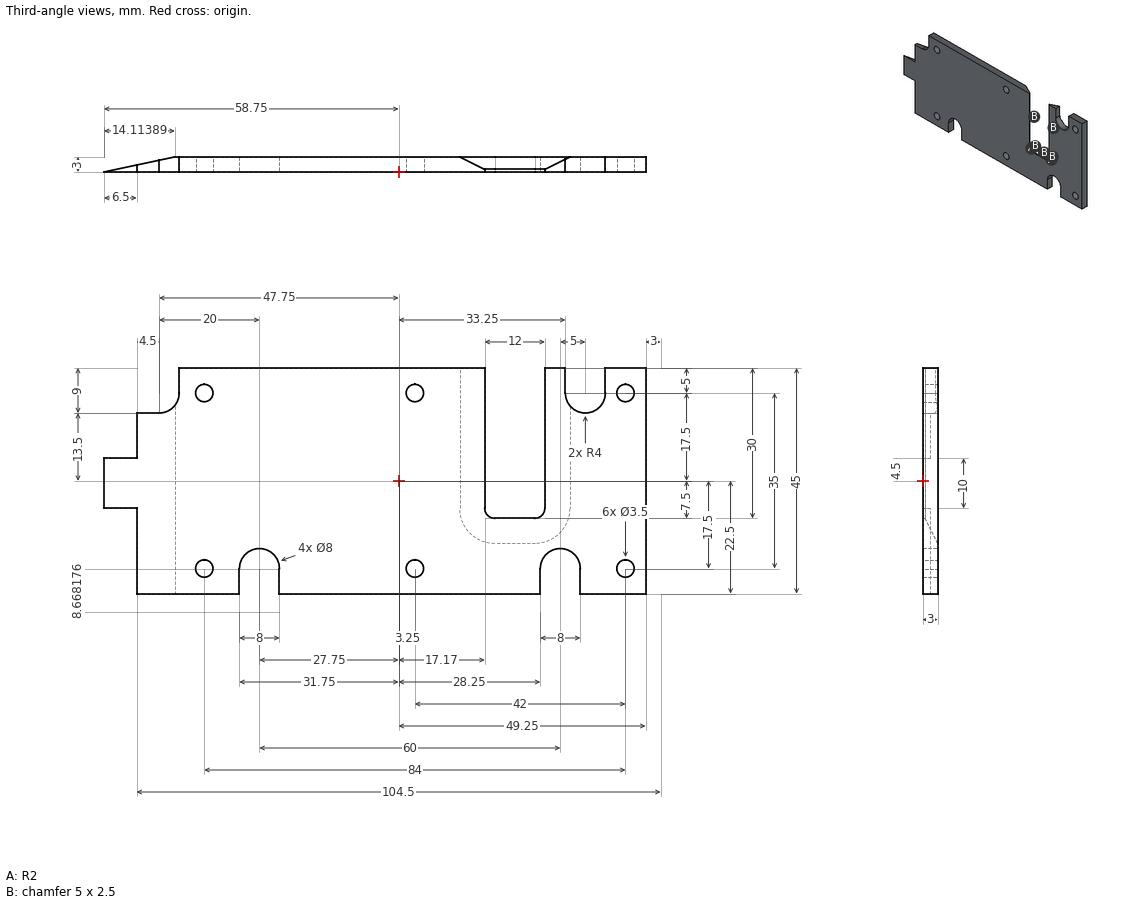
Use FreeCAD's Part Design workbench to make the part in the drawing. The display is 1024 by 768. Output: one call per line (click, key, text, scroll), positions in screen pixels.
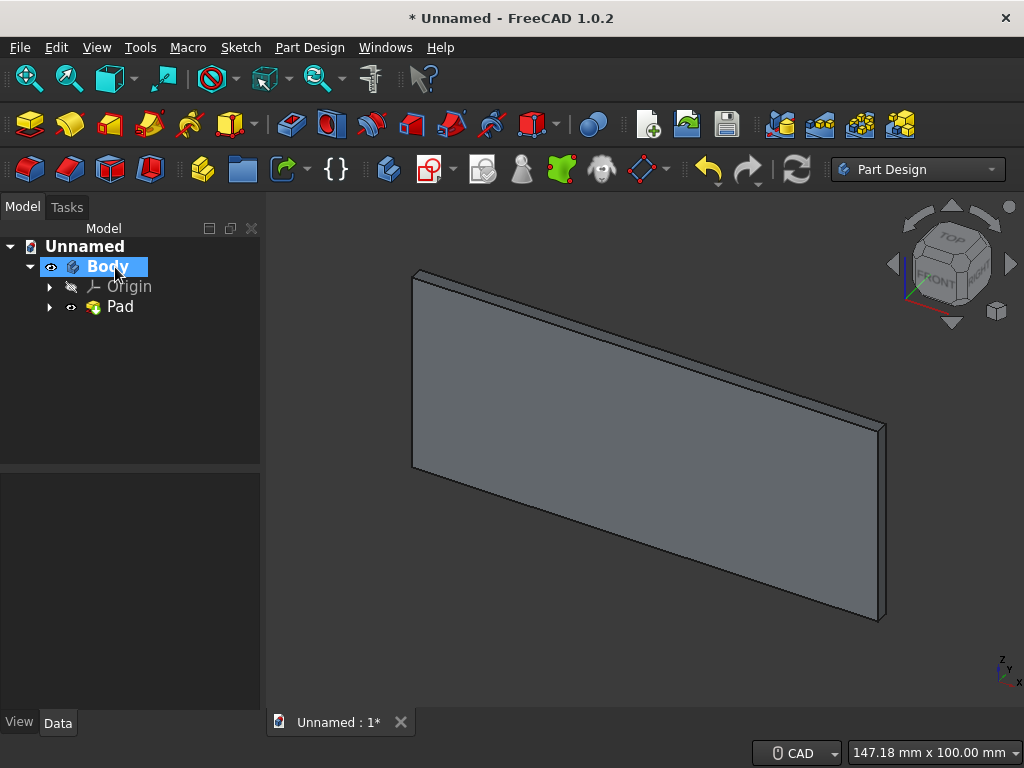
key(4)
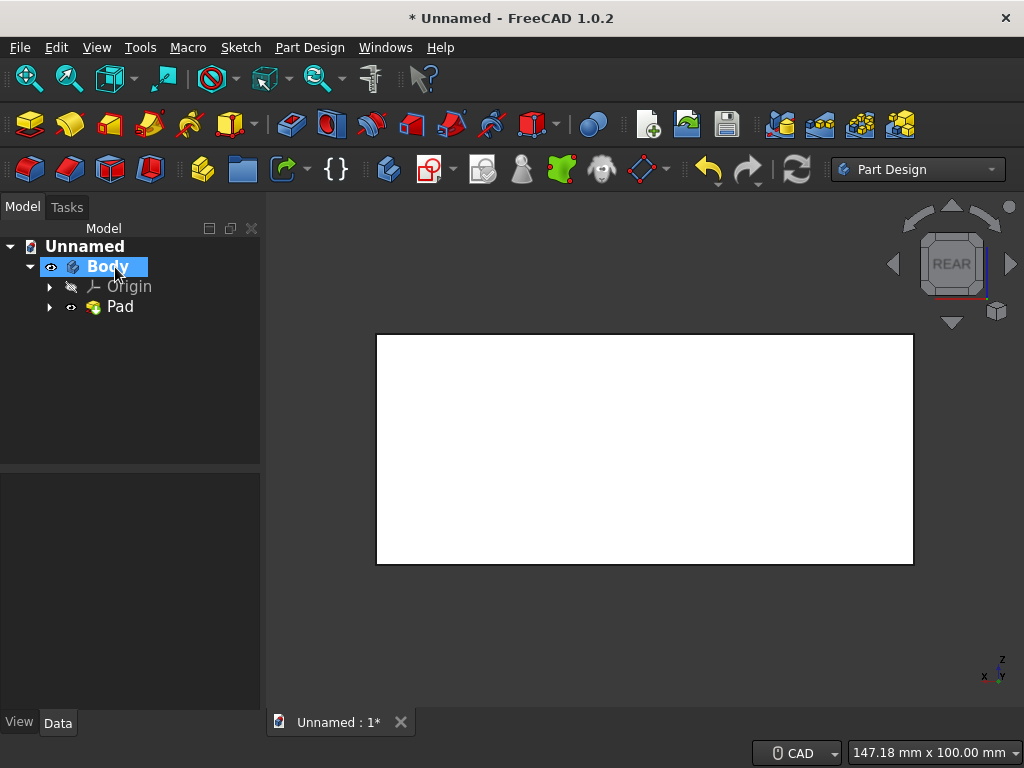
click(568, 448)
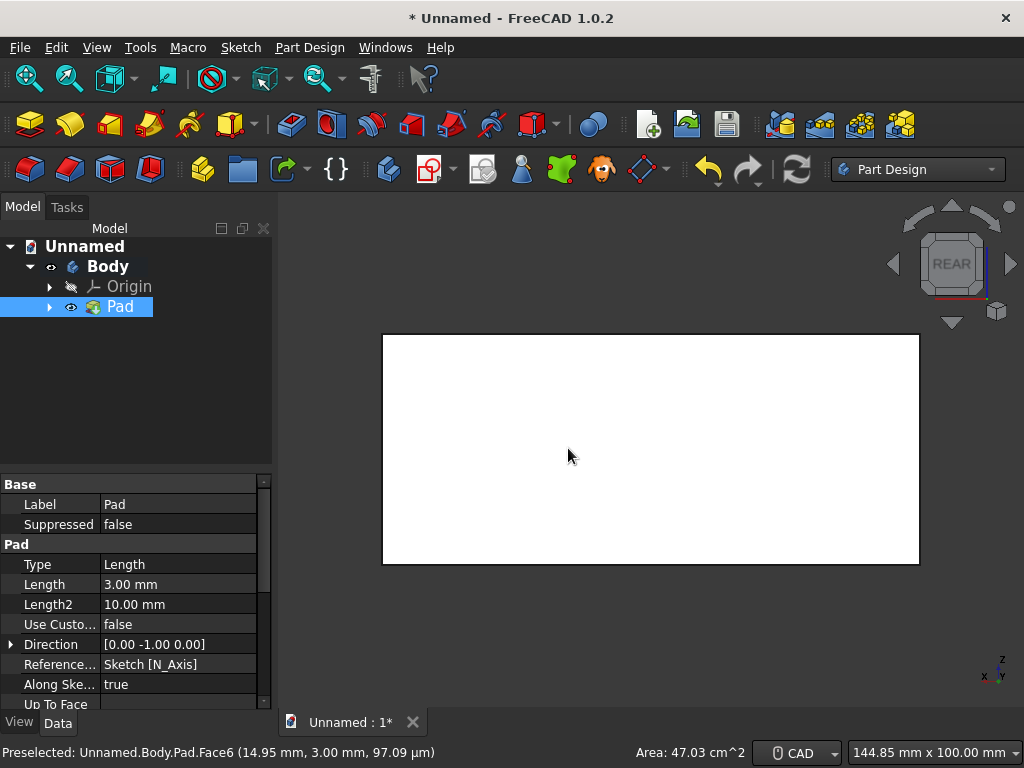
click(430, 170)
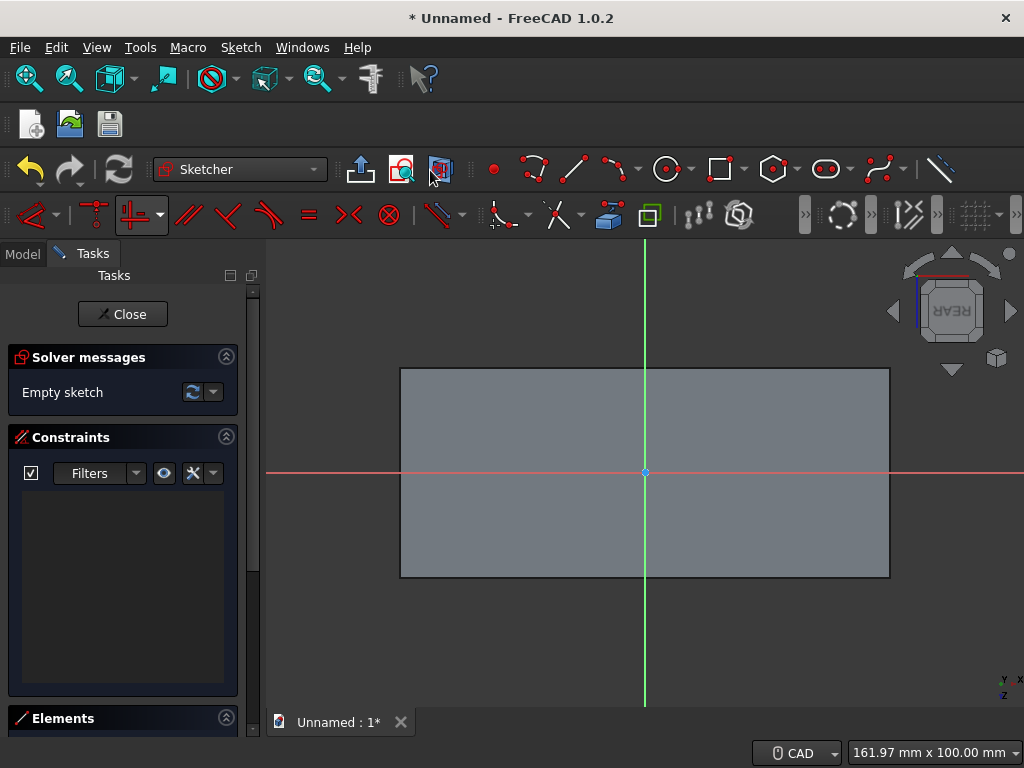
scroll(825, 537, up, 4)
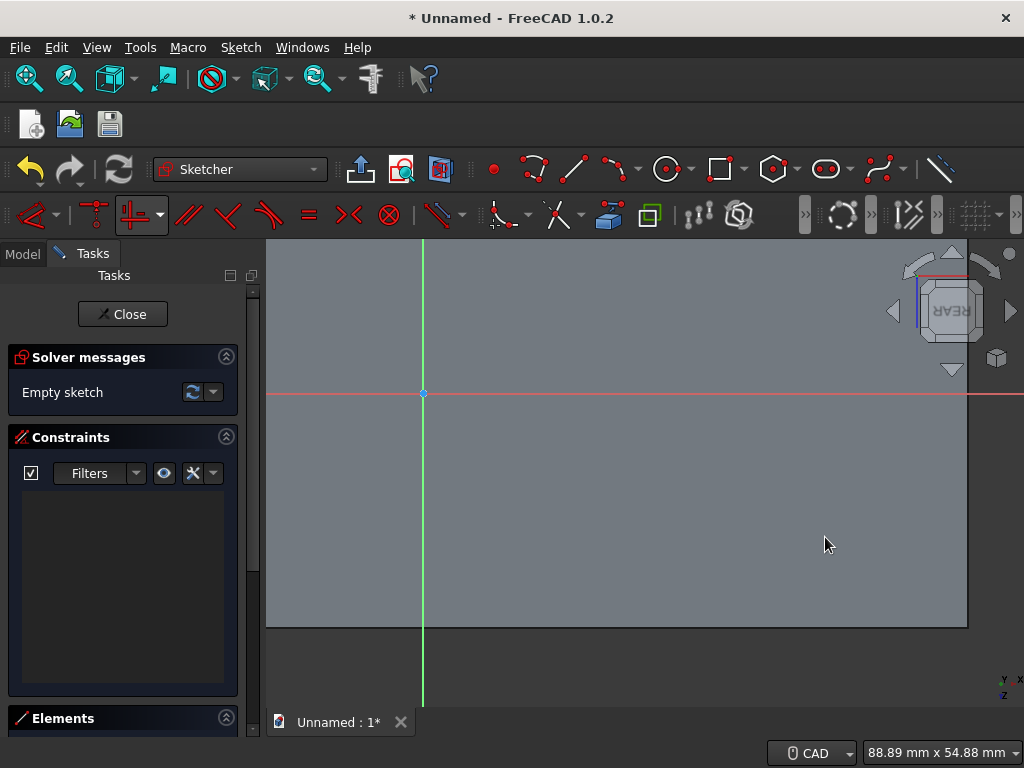
key(g)
key(r)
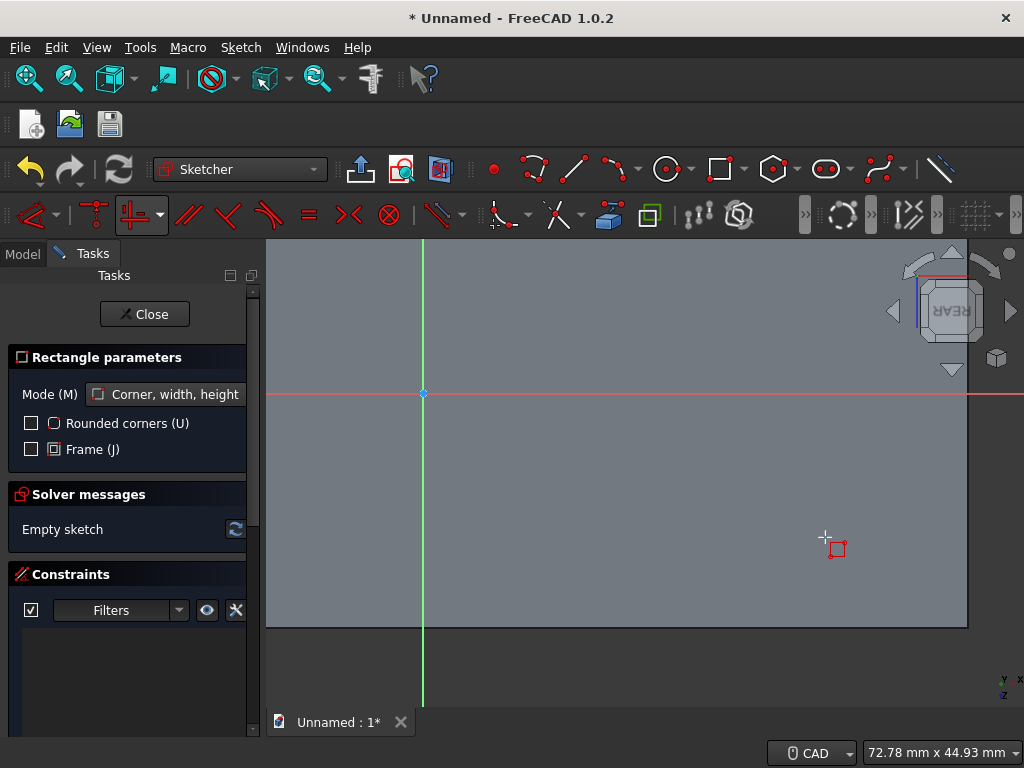
click(602, 316)
move(727, 628)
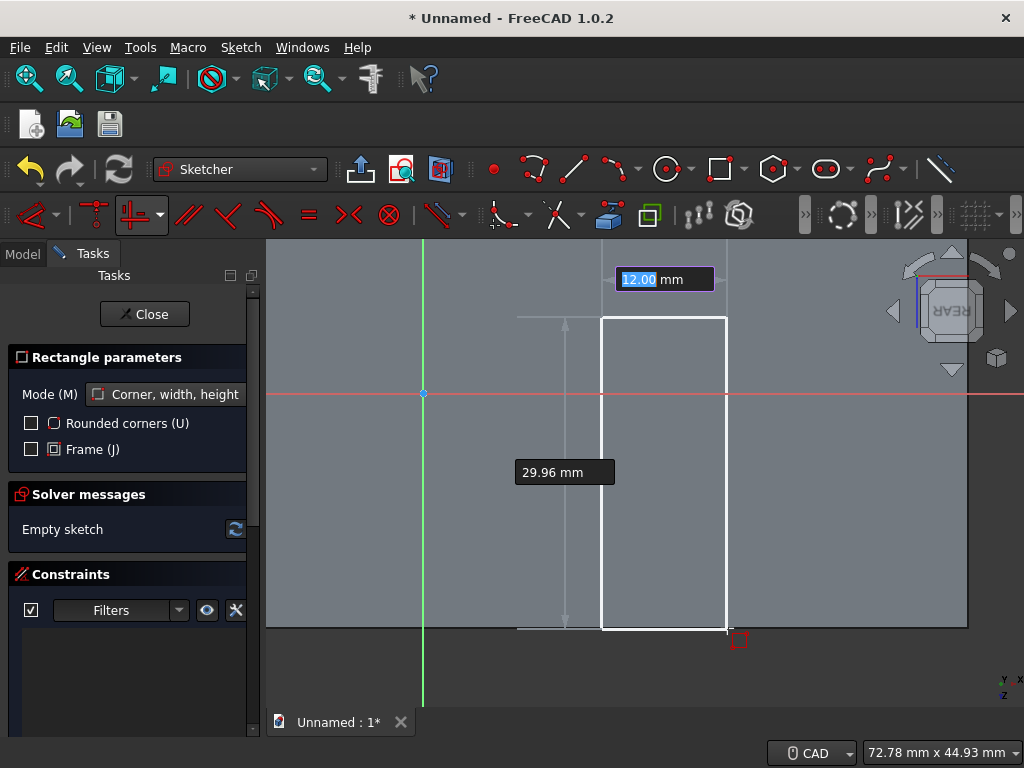
text(12)
key(Tab)
text(30)
key(Return)
key(Escape)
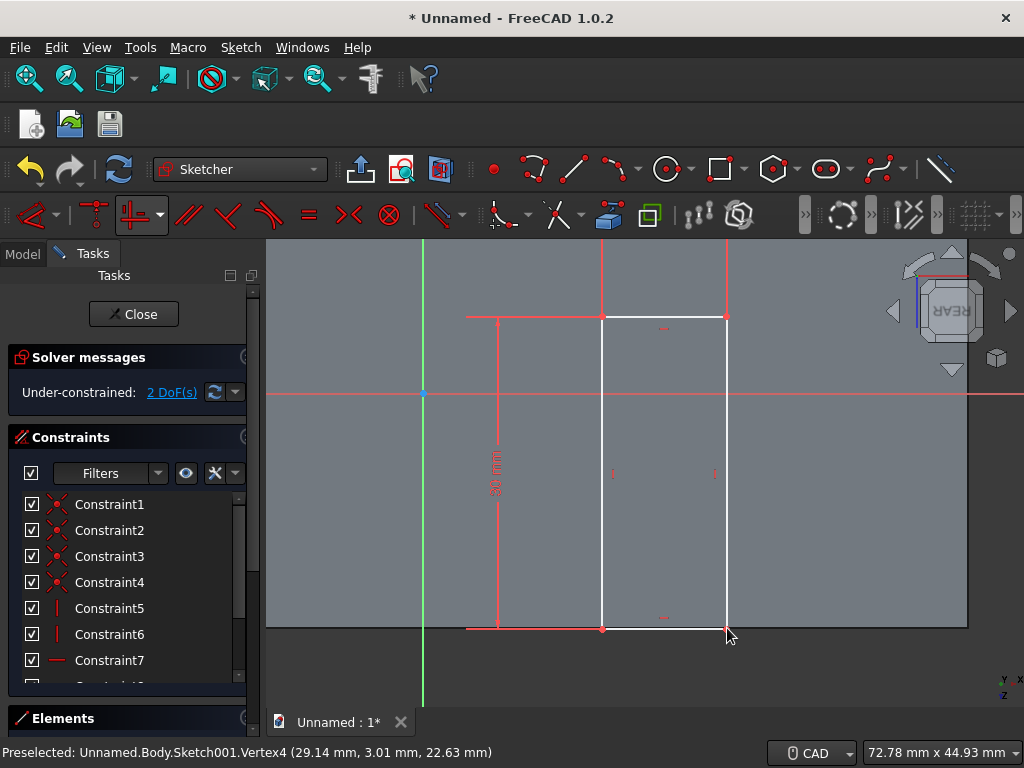
key(d)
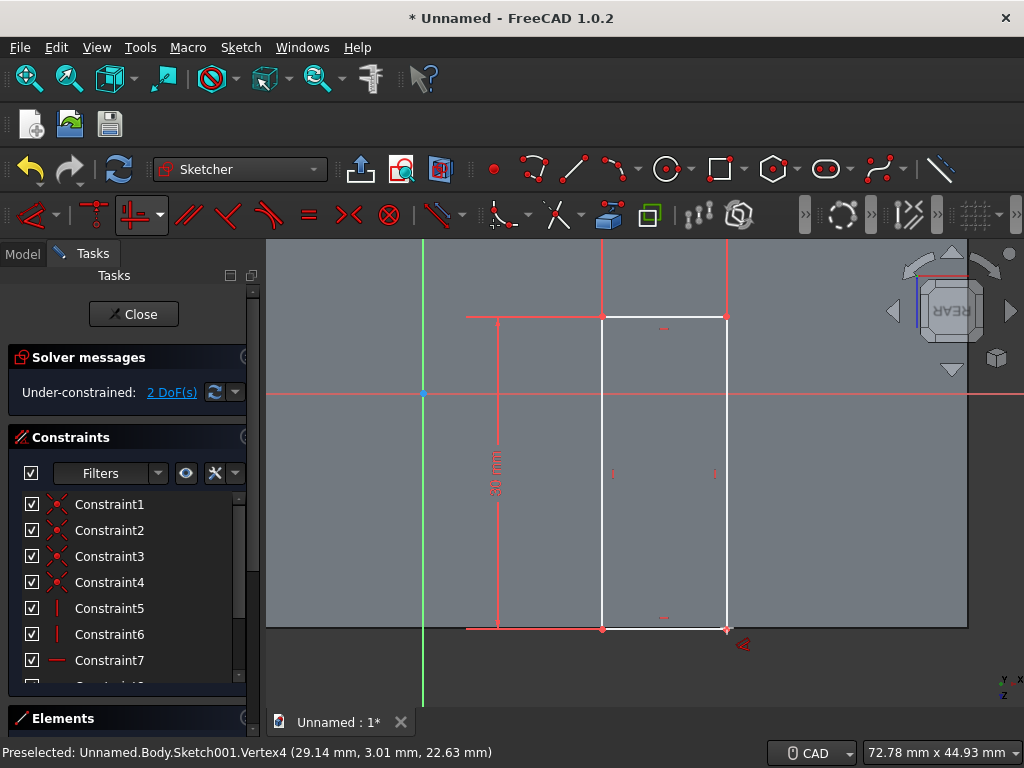
click(602, 317)
click(389, 355)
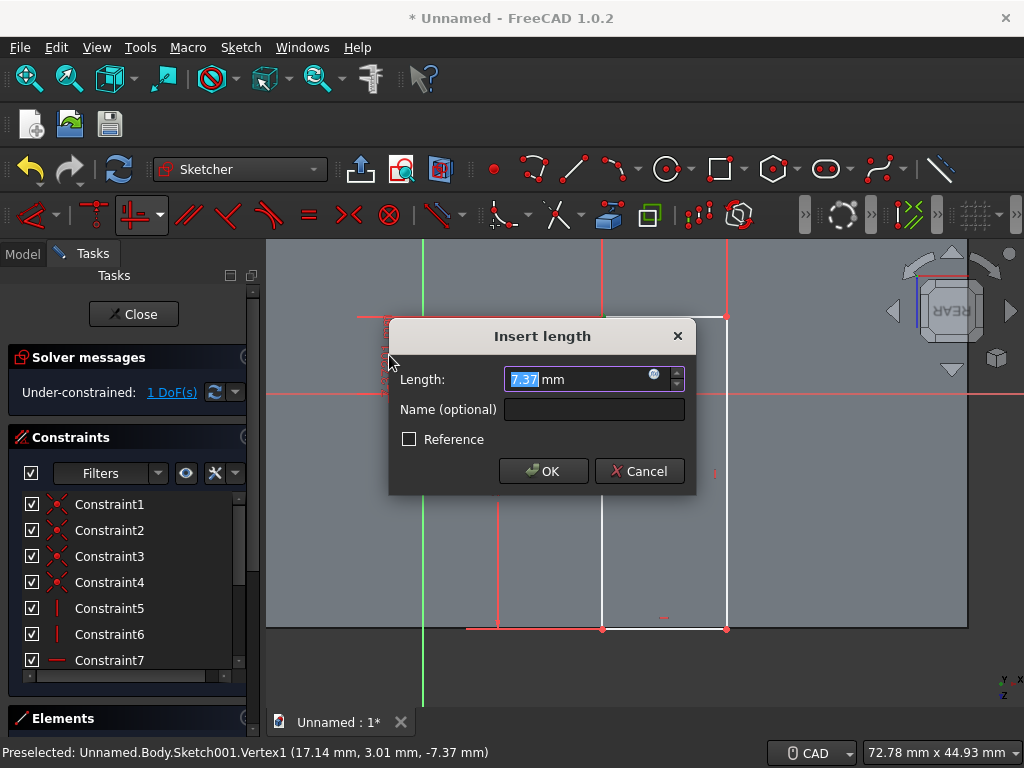
text(7.5)
key(Return)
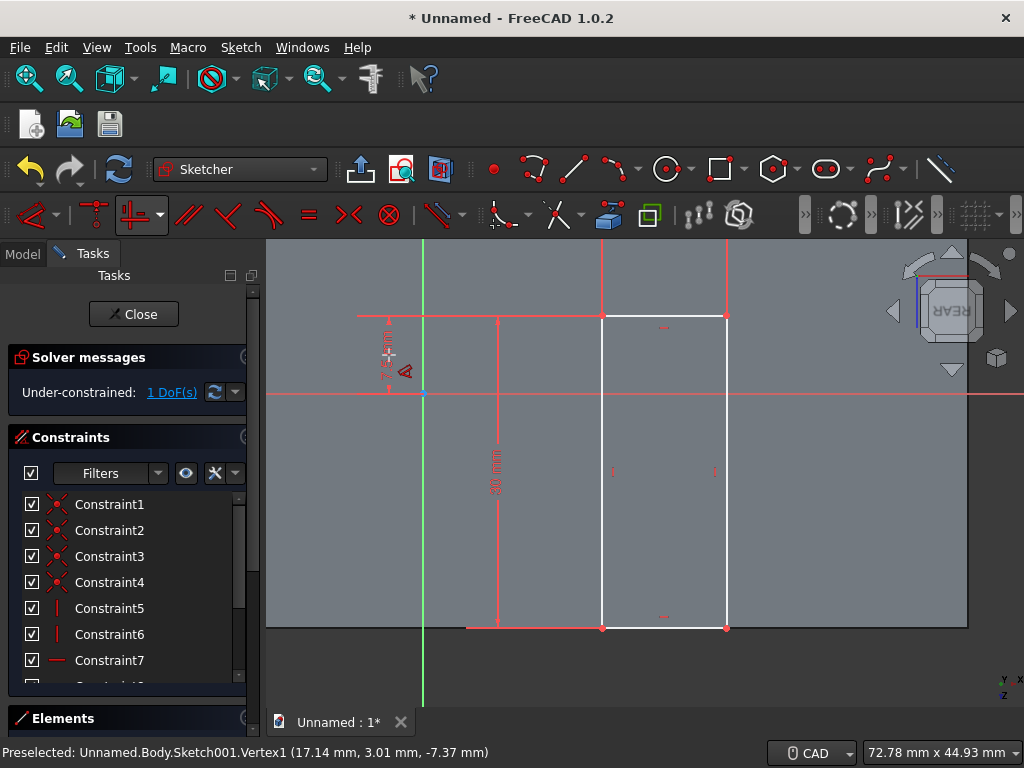
click(602, 316)
click(513, 282)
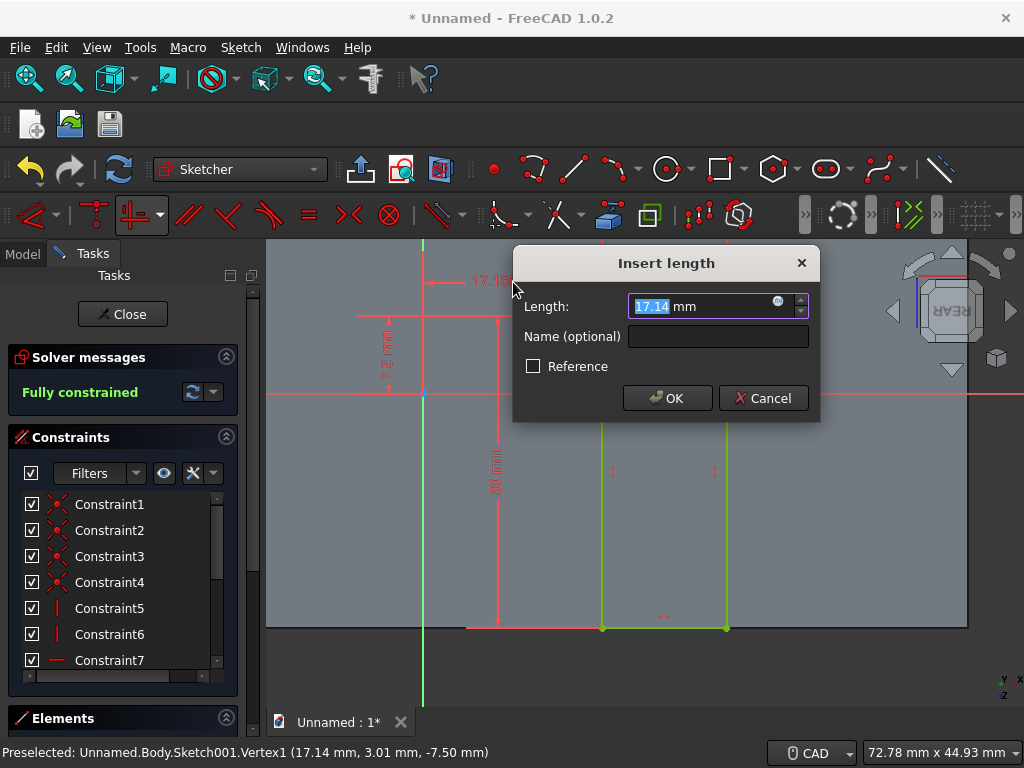
text(17.17)
key(Return)
key(Escape)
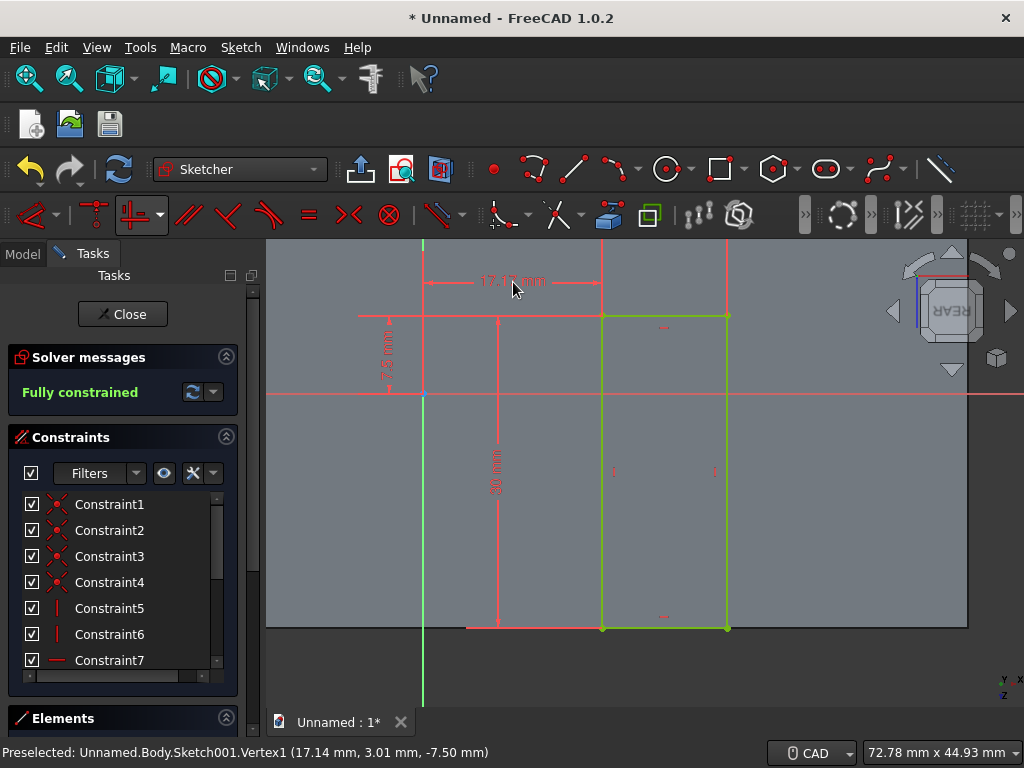
click(123, 314)